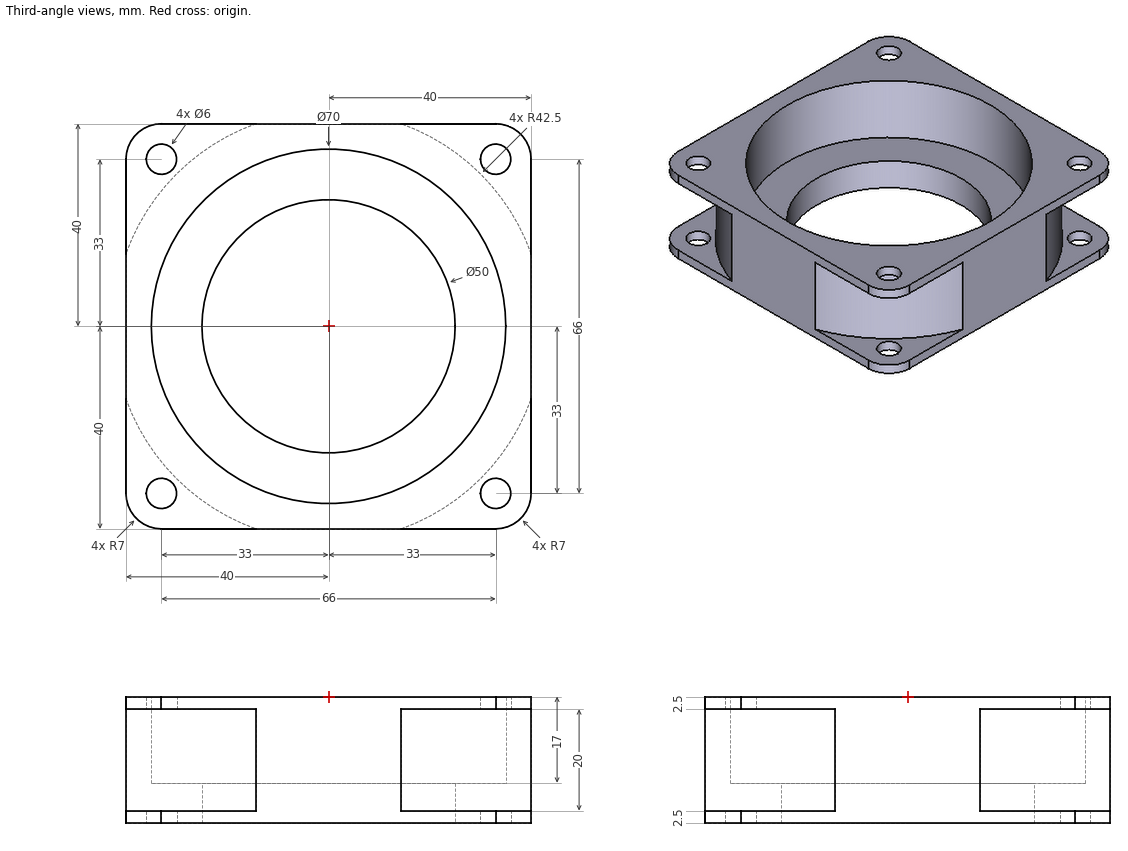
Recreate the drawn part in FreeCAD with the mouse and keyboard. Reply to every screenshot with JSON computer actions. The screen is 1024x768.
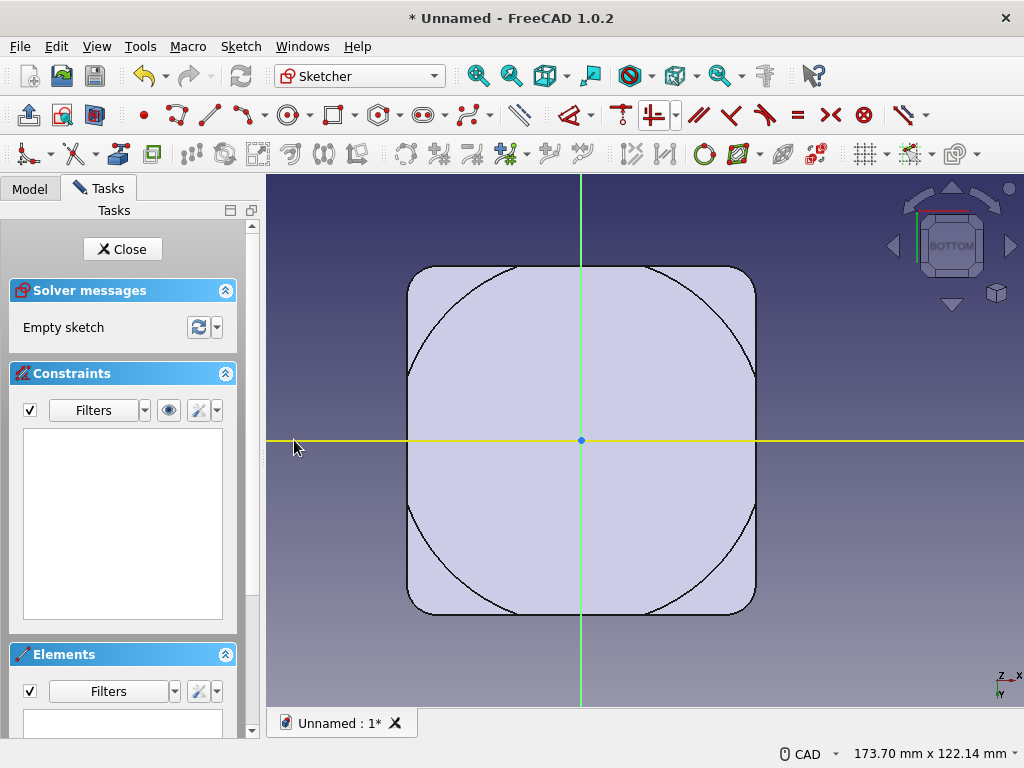
{"action": "left_click", "coordinate": [210, 116]}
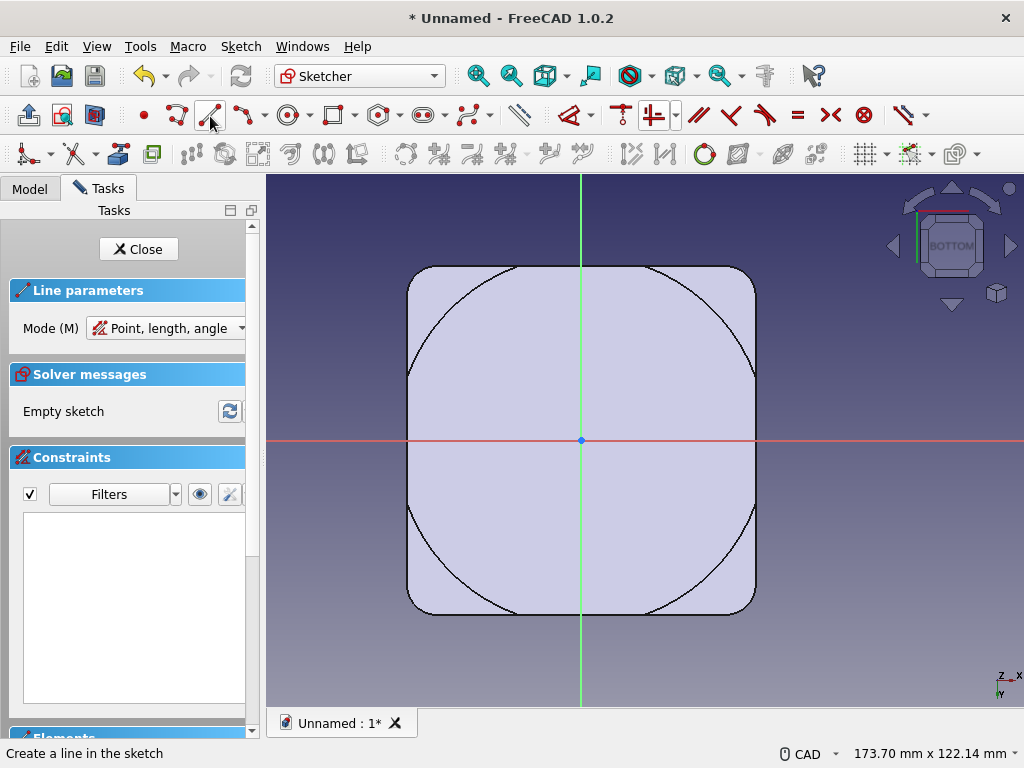
{"action": "left_click", "coordinate": [725, 266]}
{"action": "left_click", "coordinate": [437, 266]}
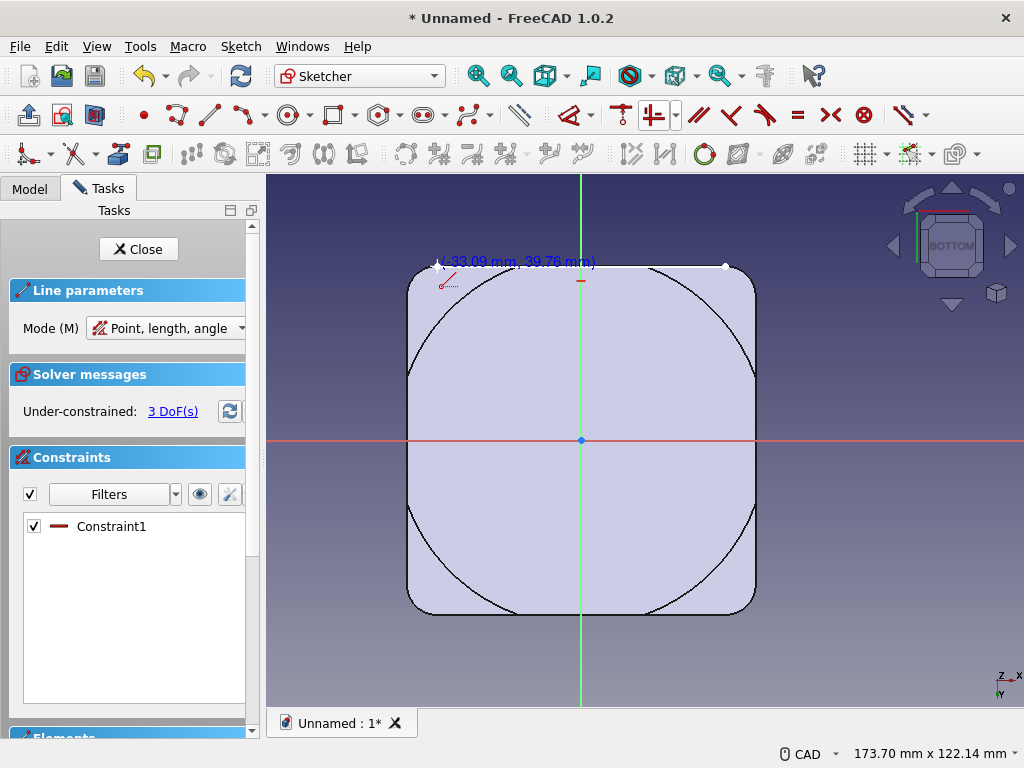
{"action": "left_click", "coordinate": [407, 296]}
{"action": "left_click", "coordinate": [407, 585]}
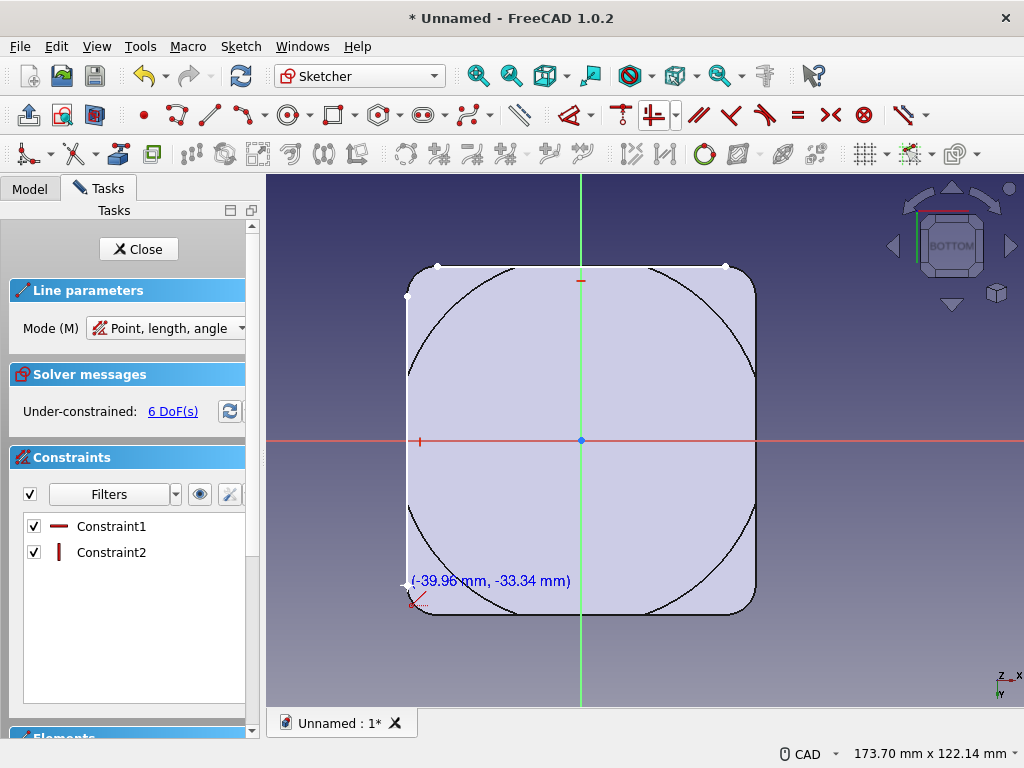
{"action": "left_click", "coordinate": [437, 615]}
{"action": "left_click", "coordinate": [725, 615]}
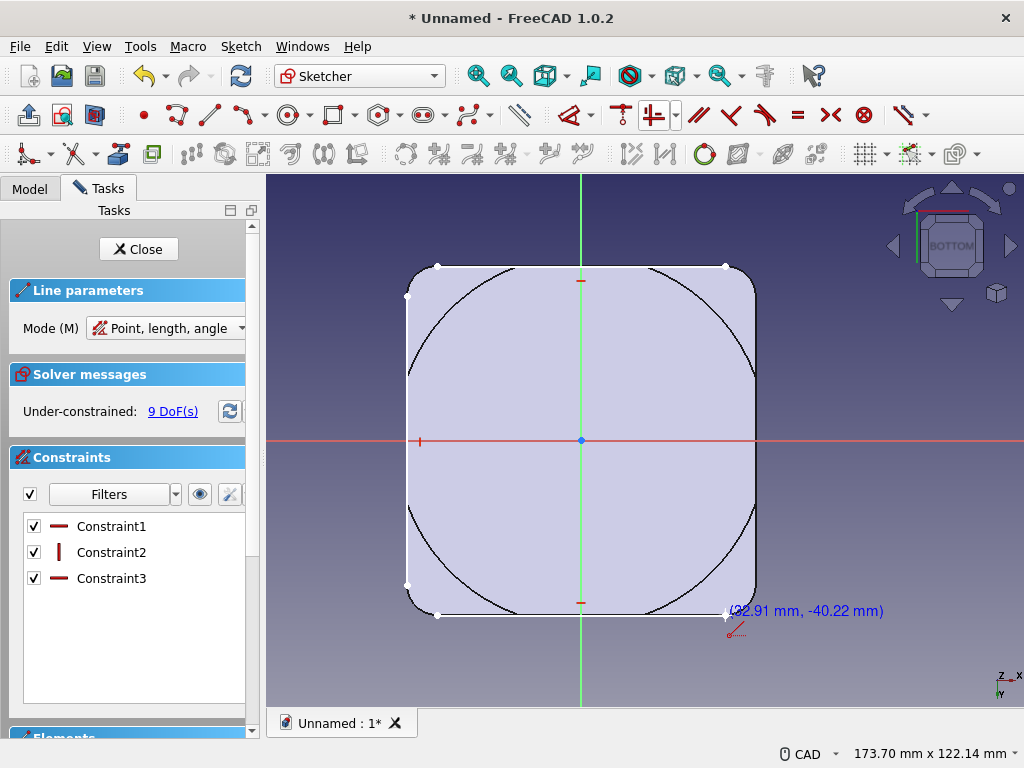
{"action": "left_click", "coordinate": [756, 585]}
{"action": "left_click", "coordinate": [756, 296]}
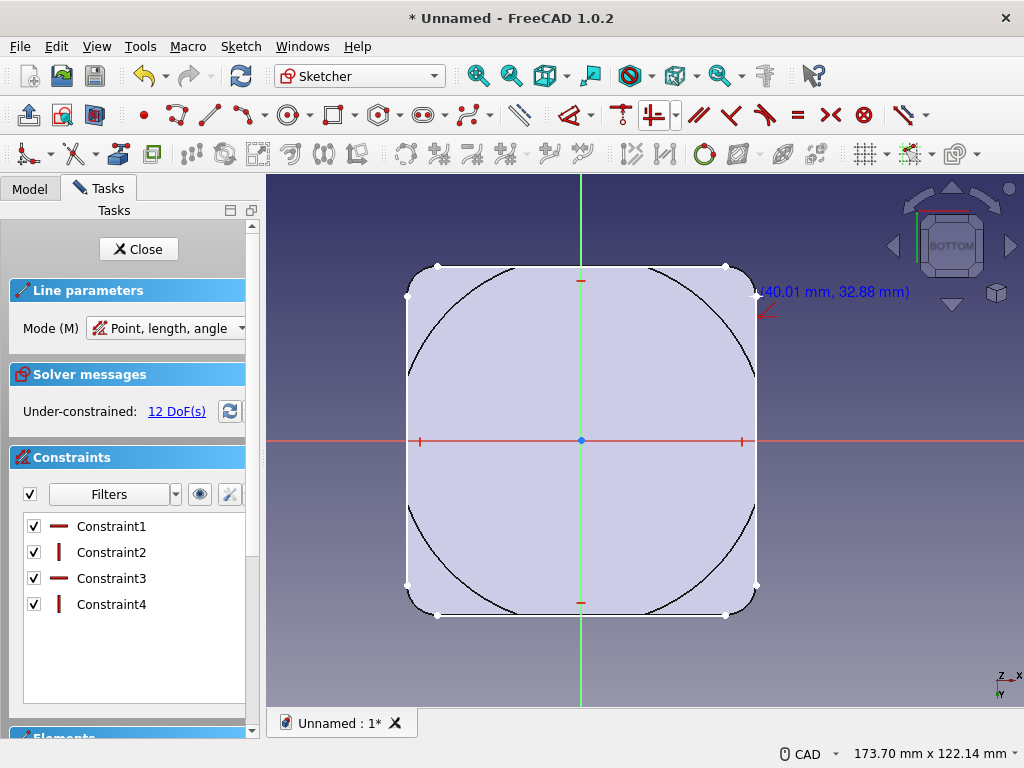
{"action": "left_click", "coordinate": [242, 116]}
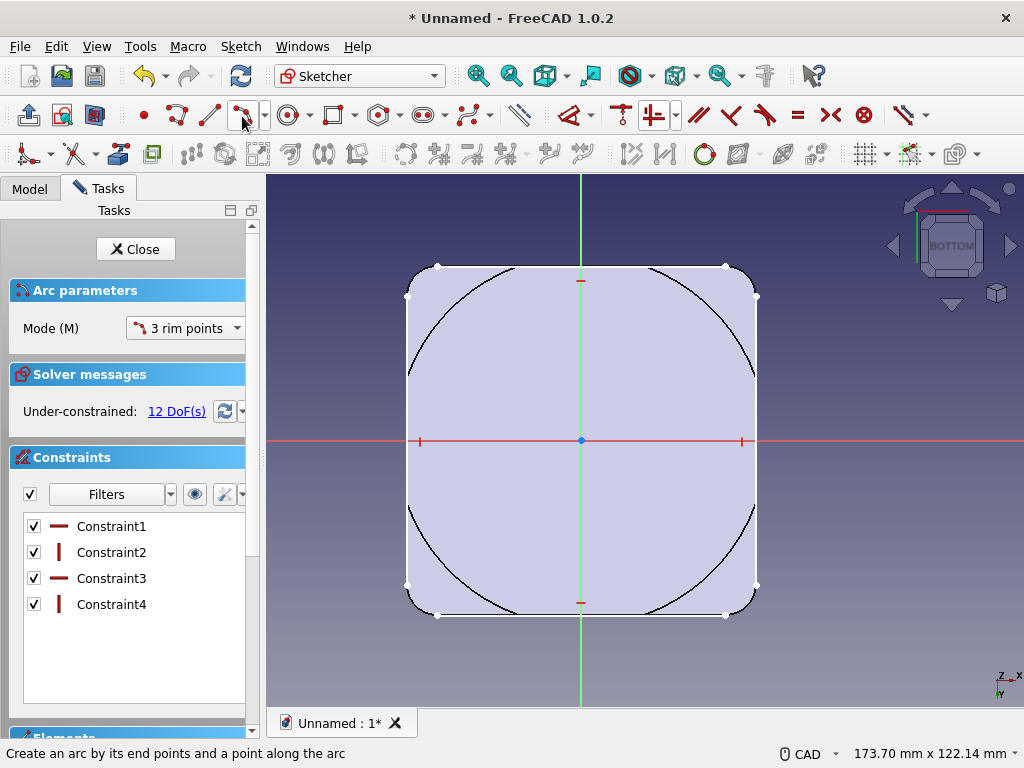
{"action": "left_click", "coordinate": [437, 267]}
{"action": "left_click", "coordinate": [407, 297]}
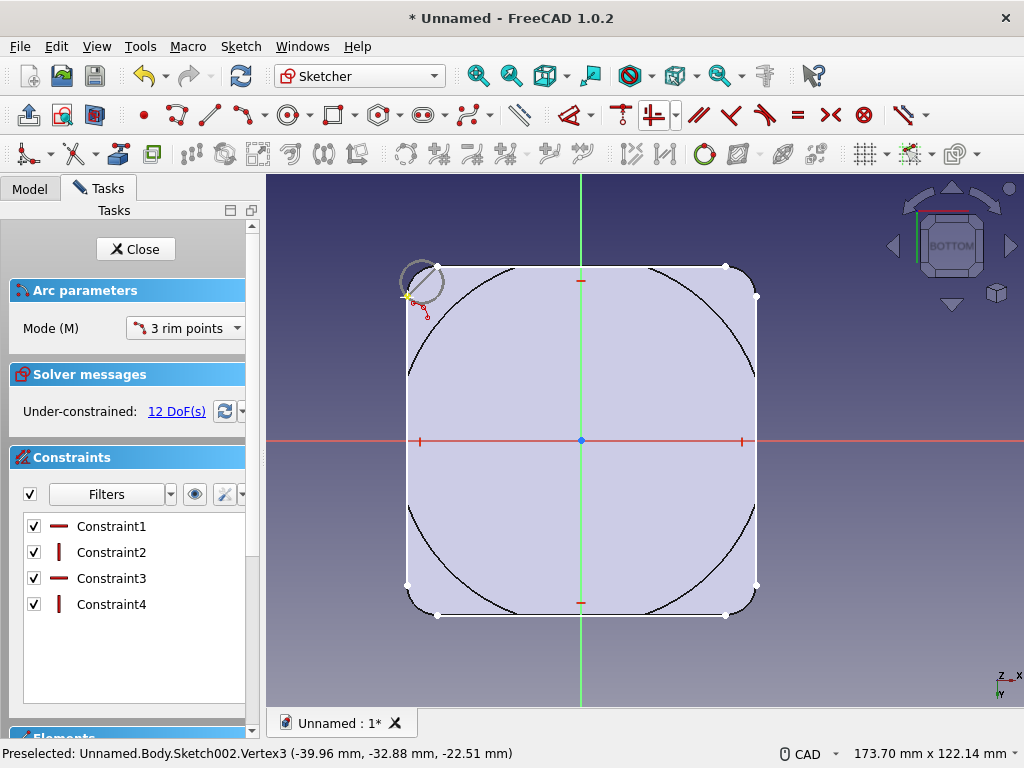
{"action": "scroll", "coordinate": [416, 275], "scroll_direction": "up", "scroll_amount": 3}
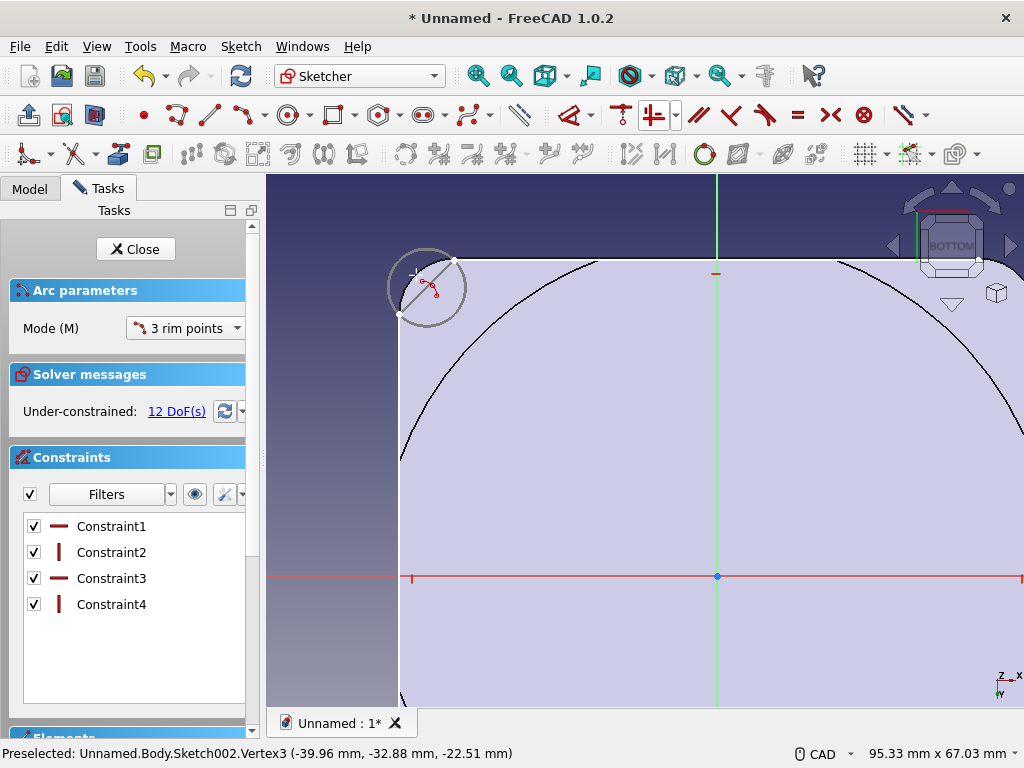
{"action": "left_click", "coordinate": [415, 275]}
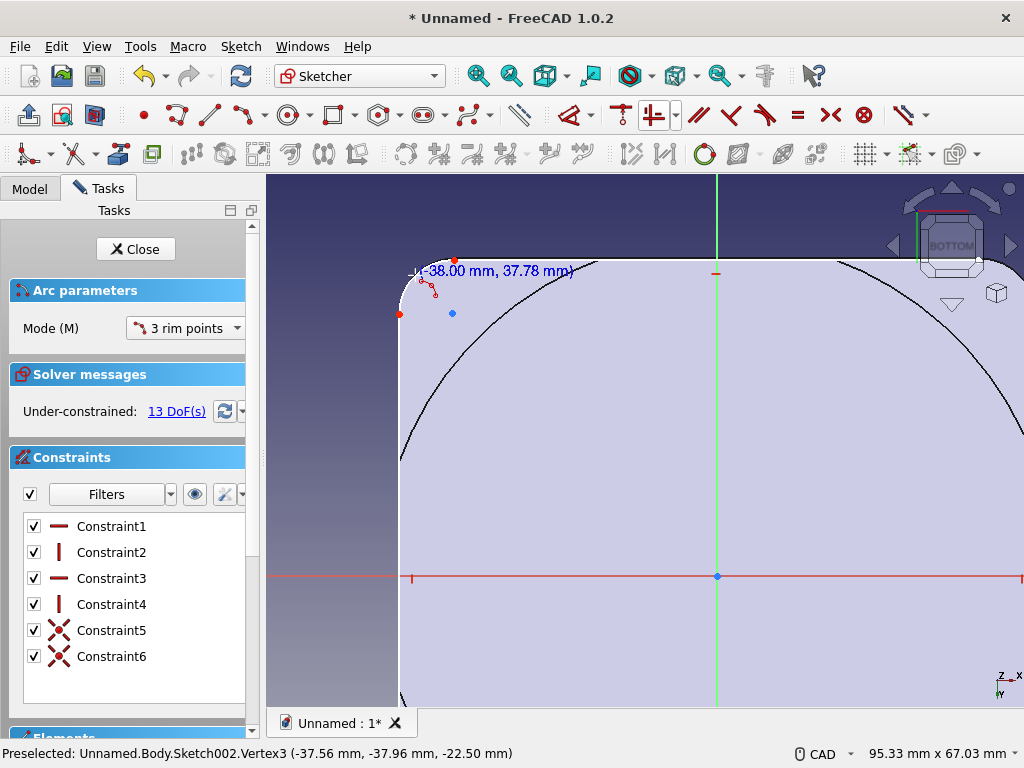
{"action": "scroll", "coordinate": [405, 275], "scroll_direction": "down", "scroll_amount": 3}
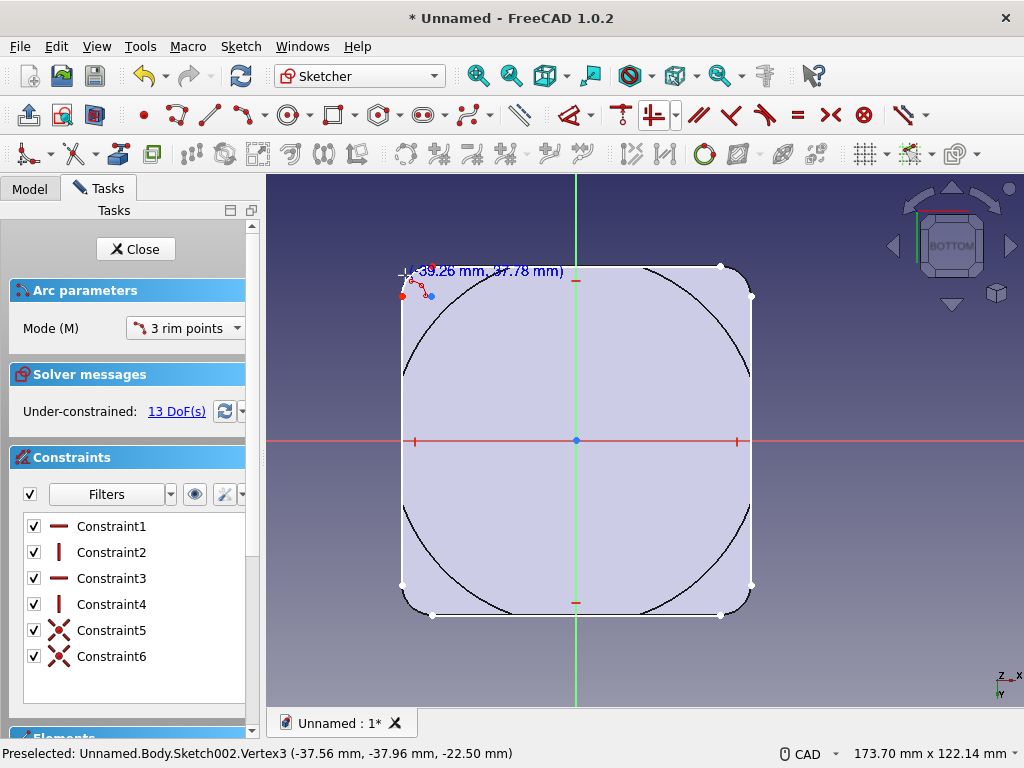
{"action": "left_click", "coordinate": [402, 586]}
{"action": "left_click", "coordinate": [432, 616]}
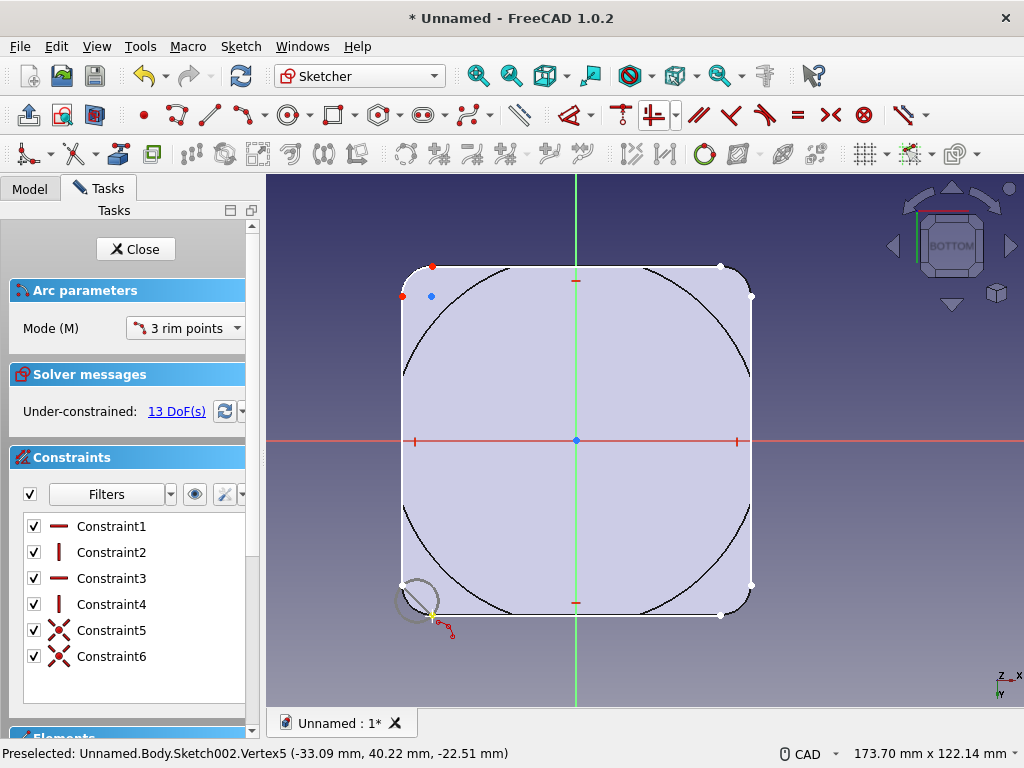
{"action": "scroll", "coordinate": [411, 606], "scroll_direction": "up", "scroll_amount": 3}